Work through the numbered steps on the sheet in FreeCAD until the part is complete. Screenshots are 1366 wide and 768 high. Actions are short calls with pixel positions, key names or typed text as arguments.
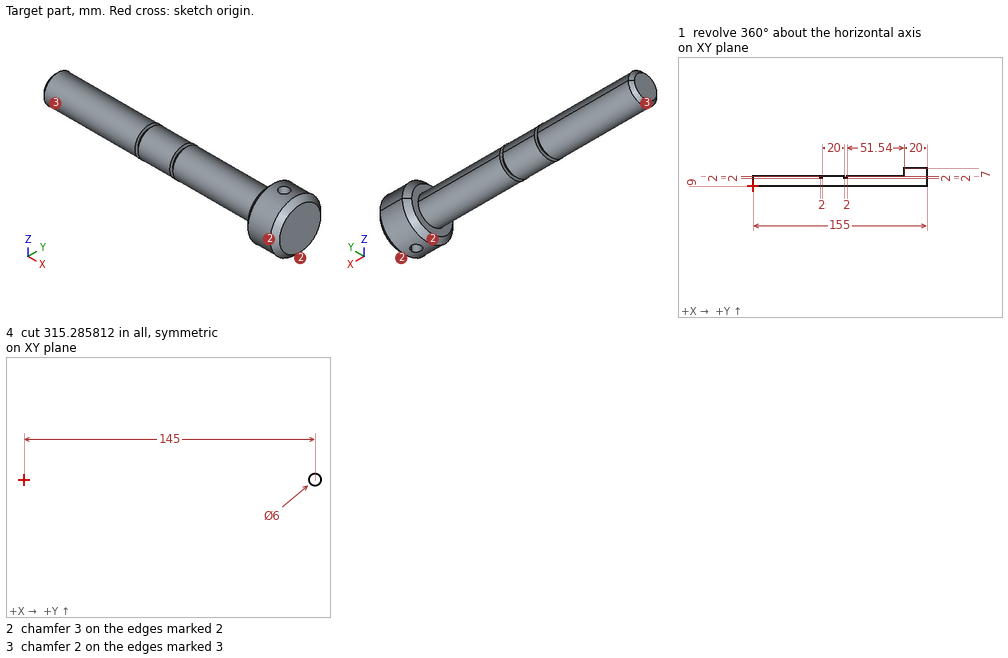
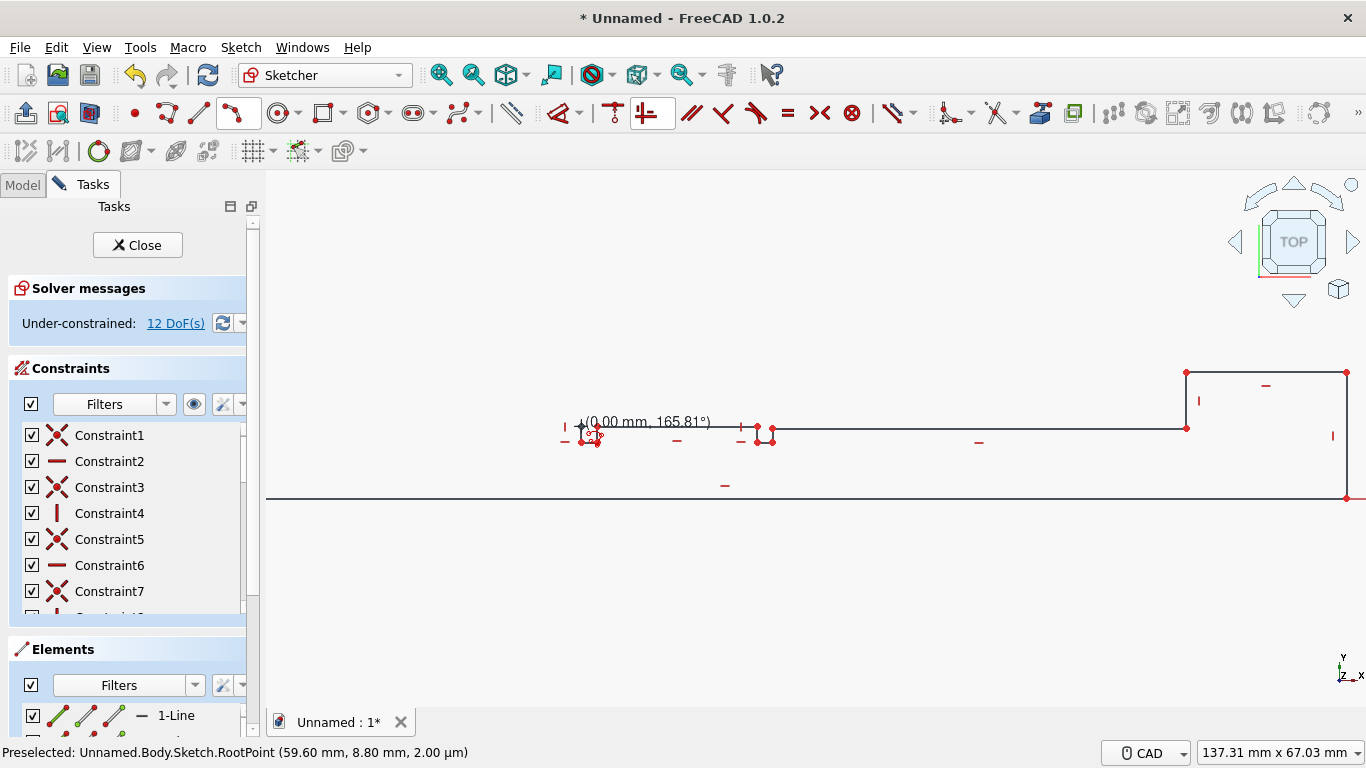
scroll(774, 443, down, 3)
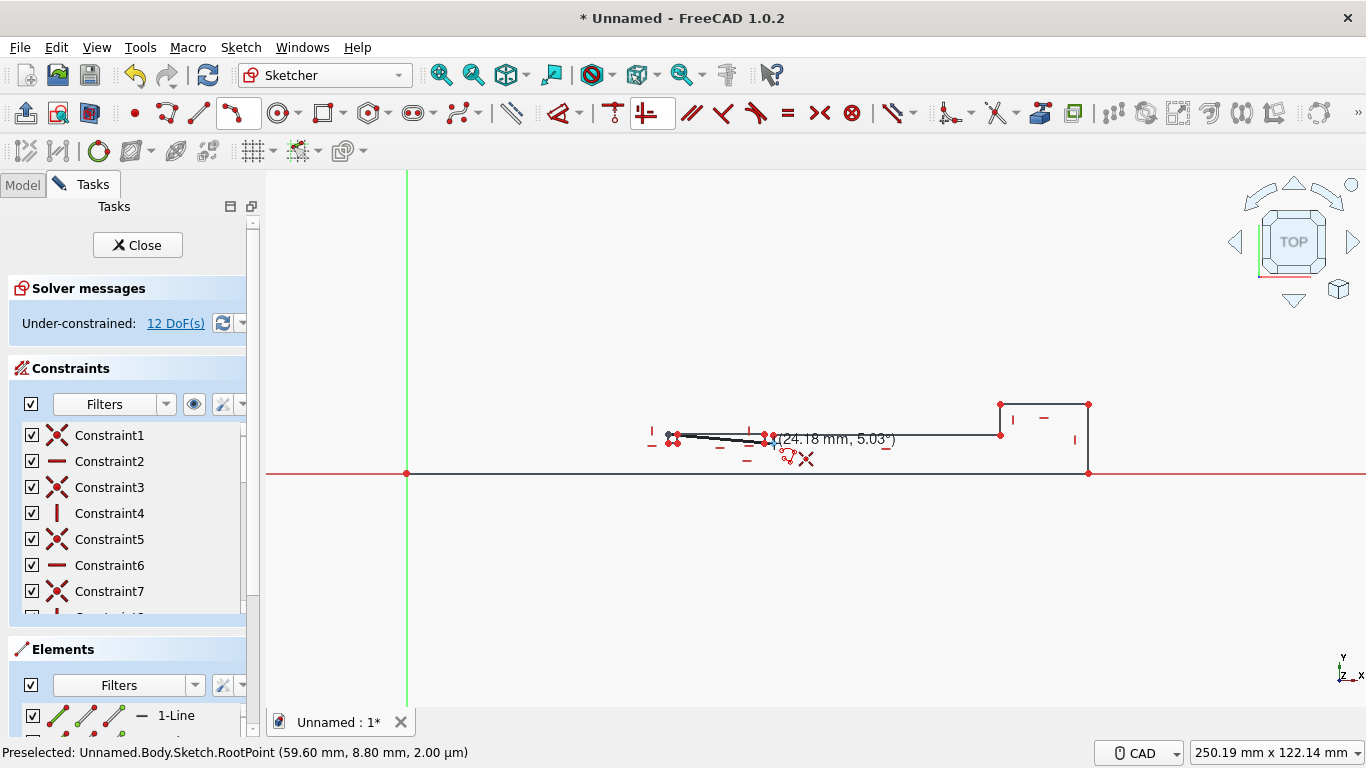
click(416, 434)
click(407, 474)
key(Escape)
key(Escape)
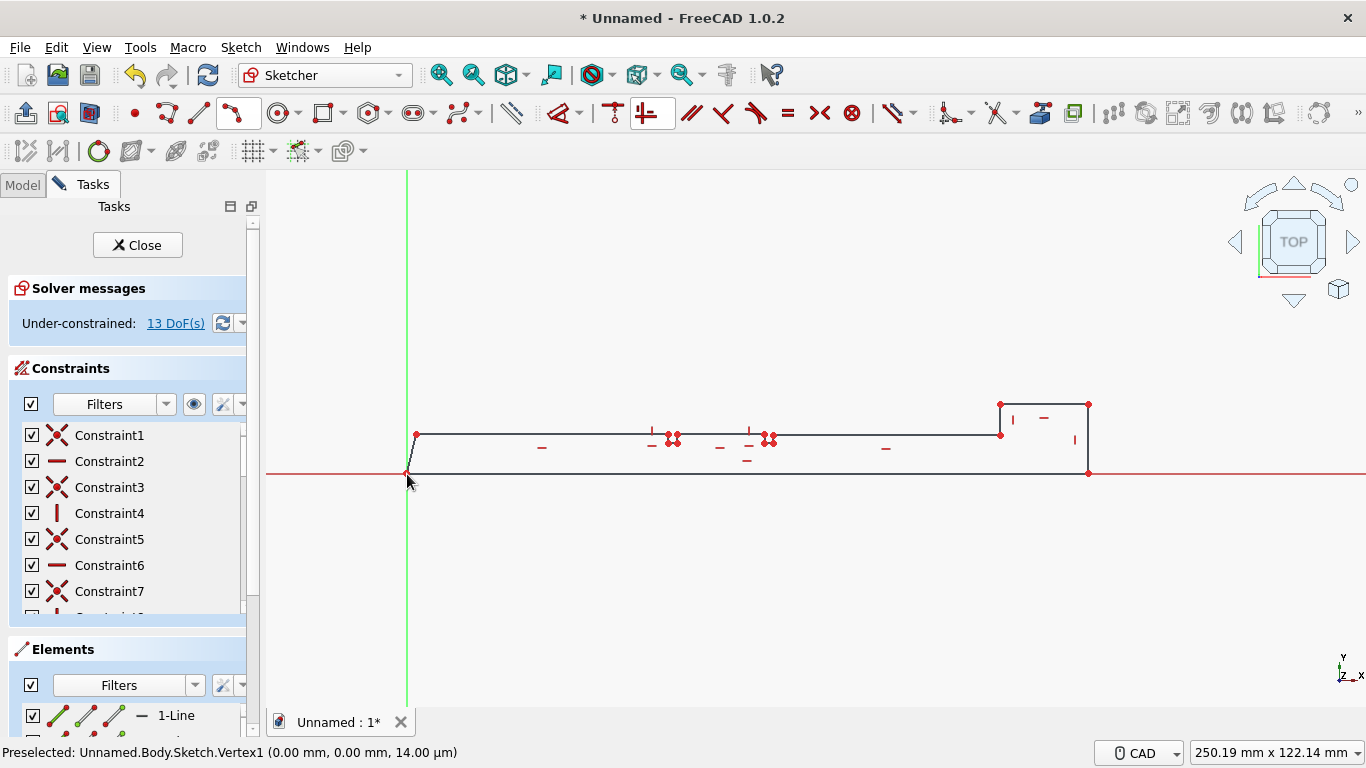
click(410, 462)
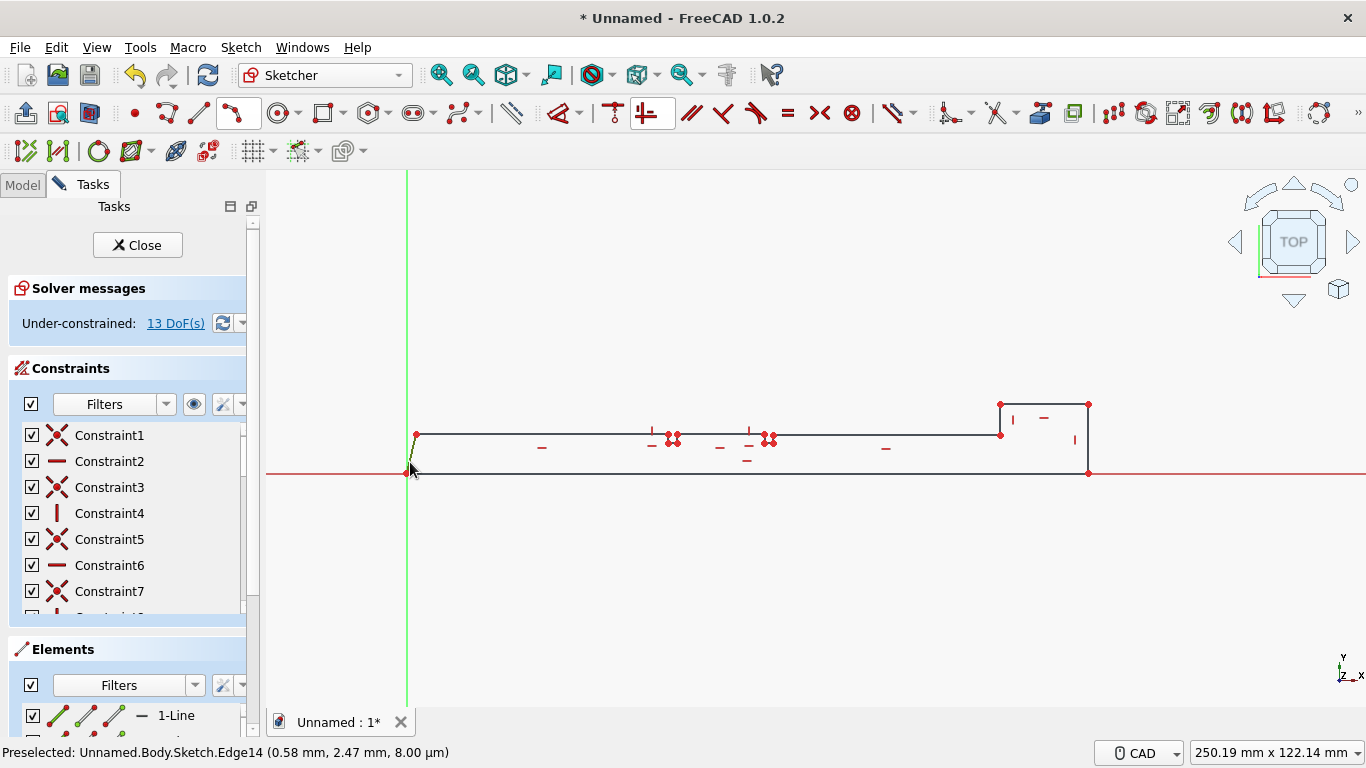
click(670, 114)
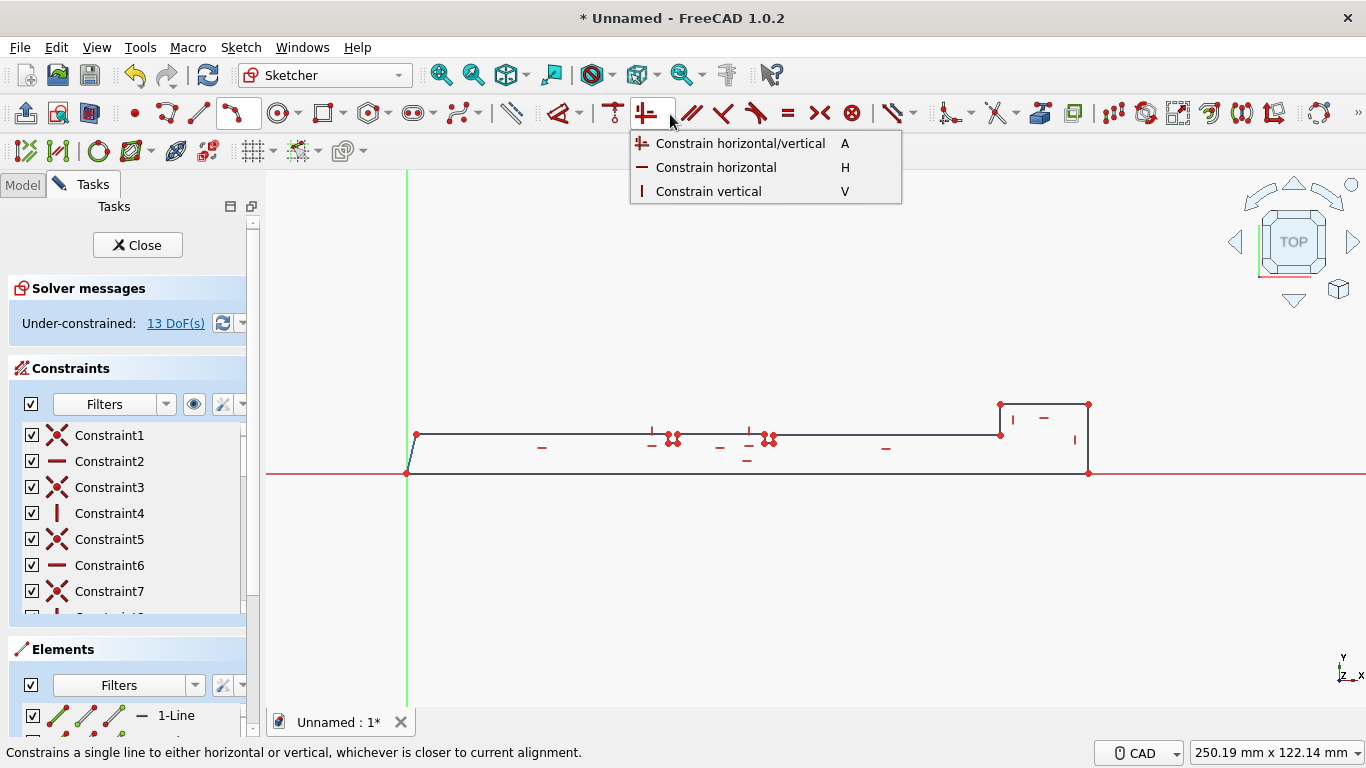
click(766, 191)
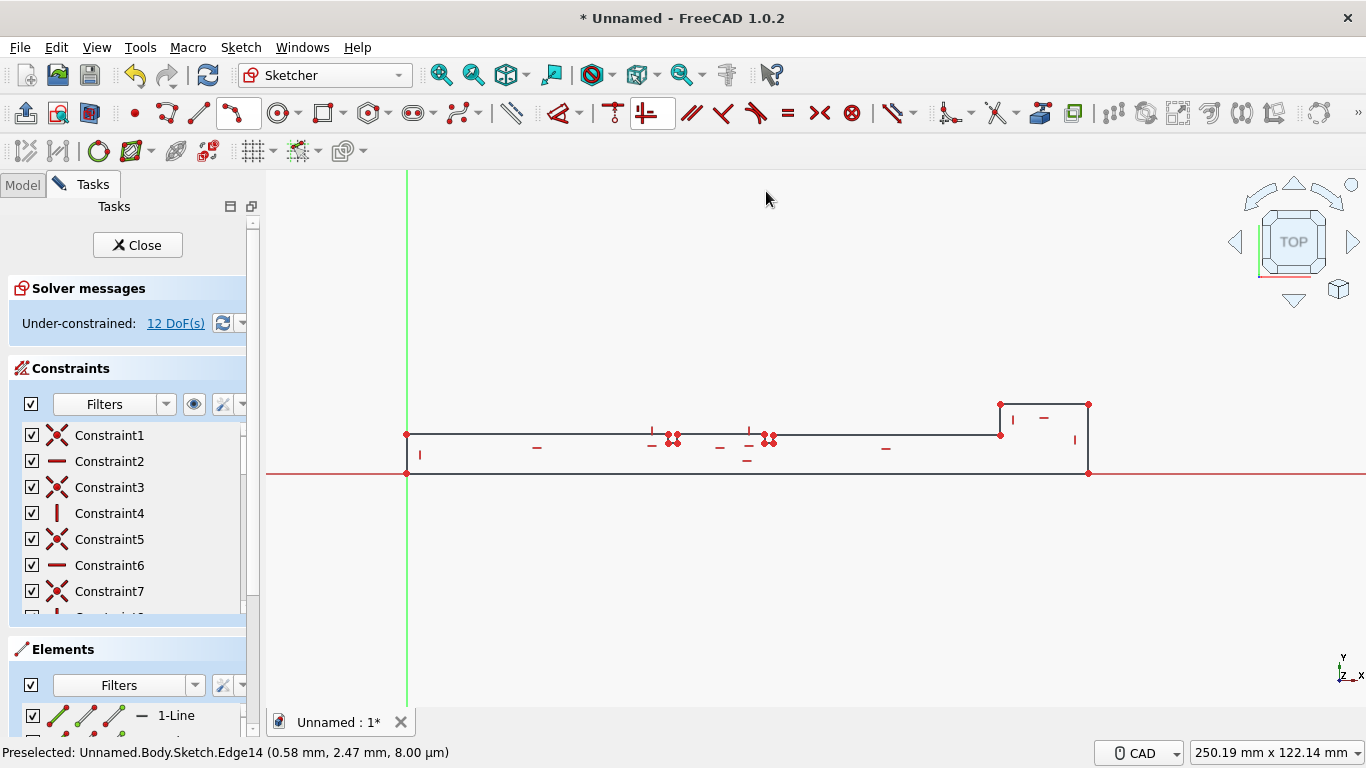
click(558, 114)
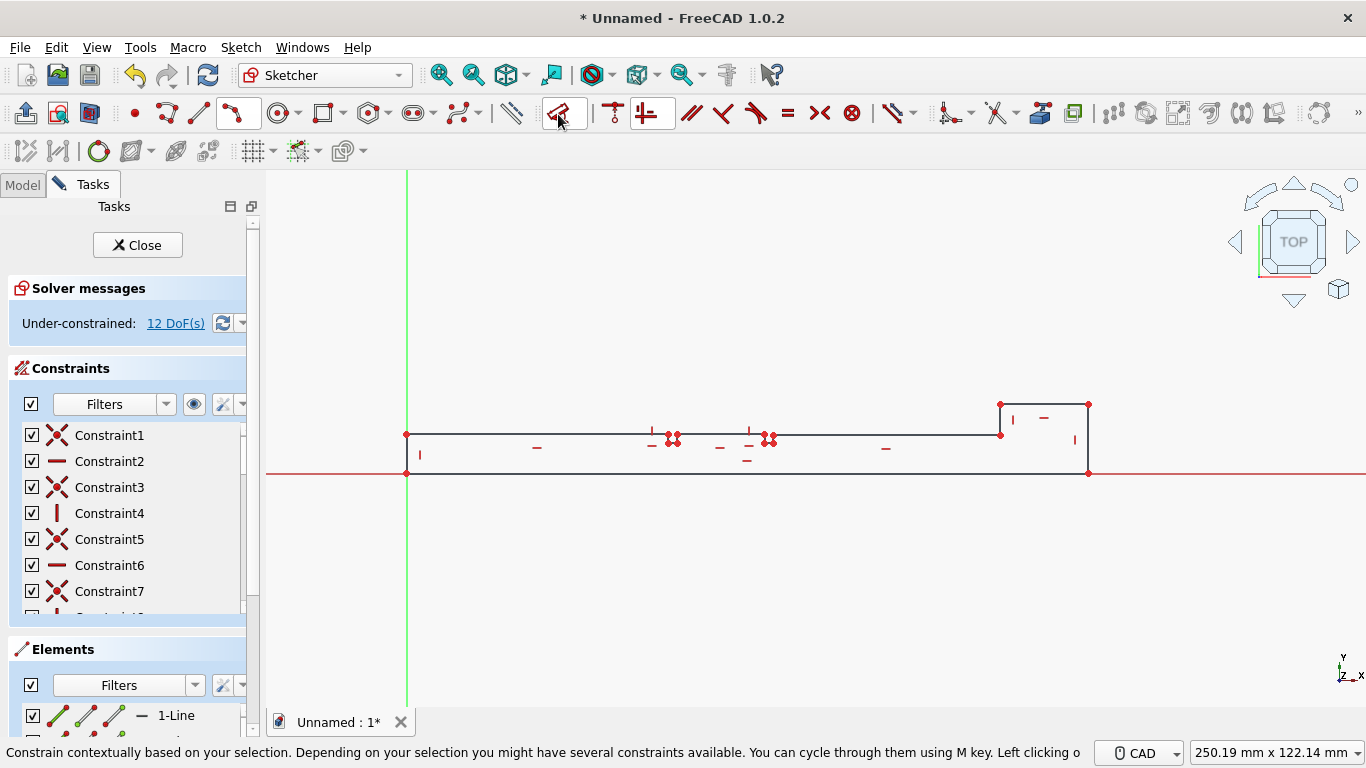
scroll(1000, 414, up, 2)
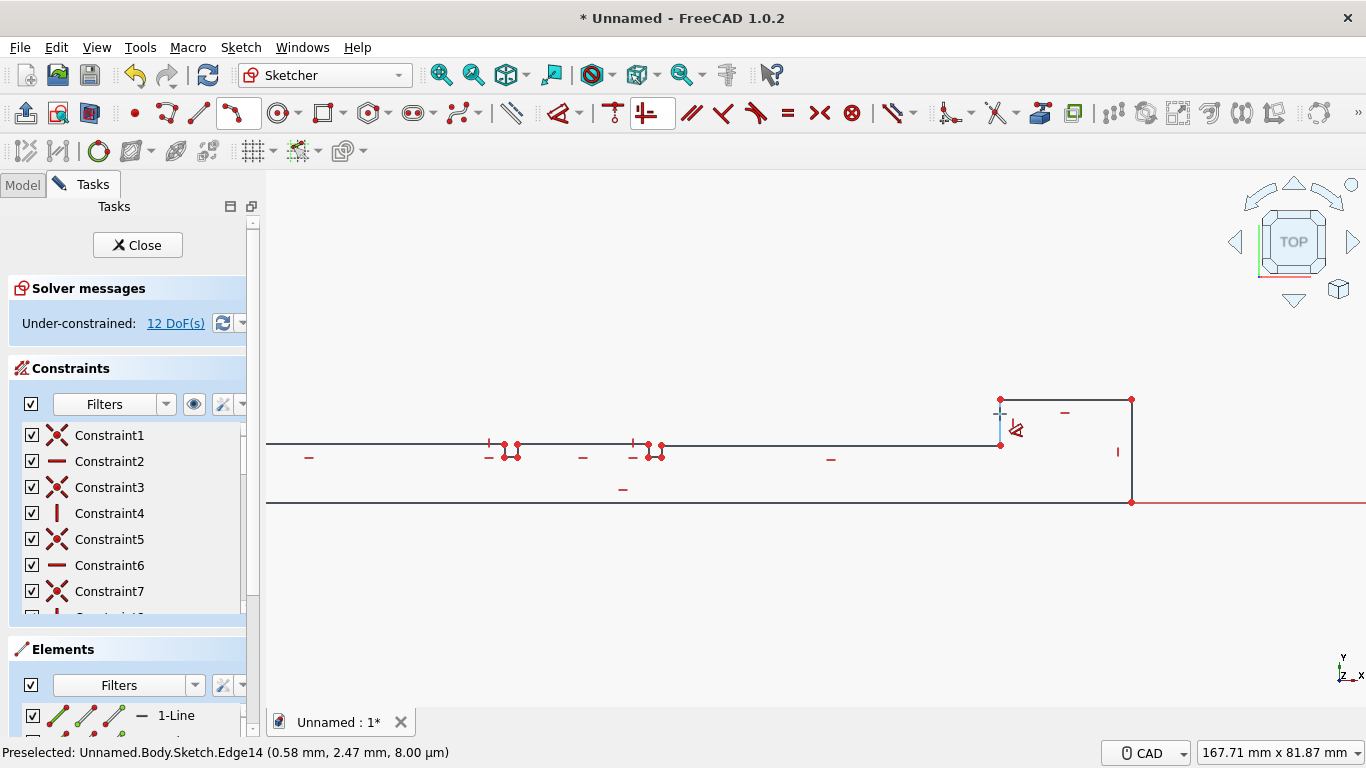
click(1000, 413)
click(1034, 423)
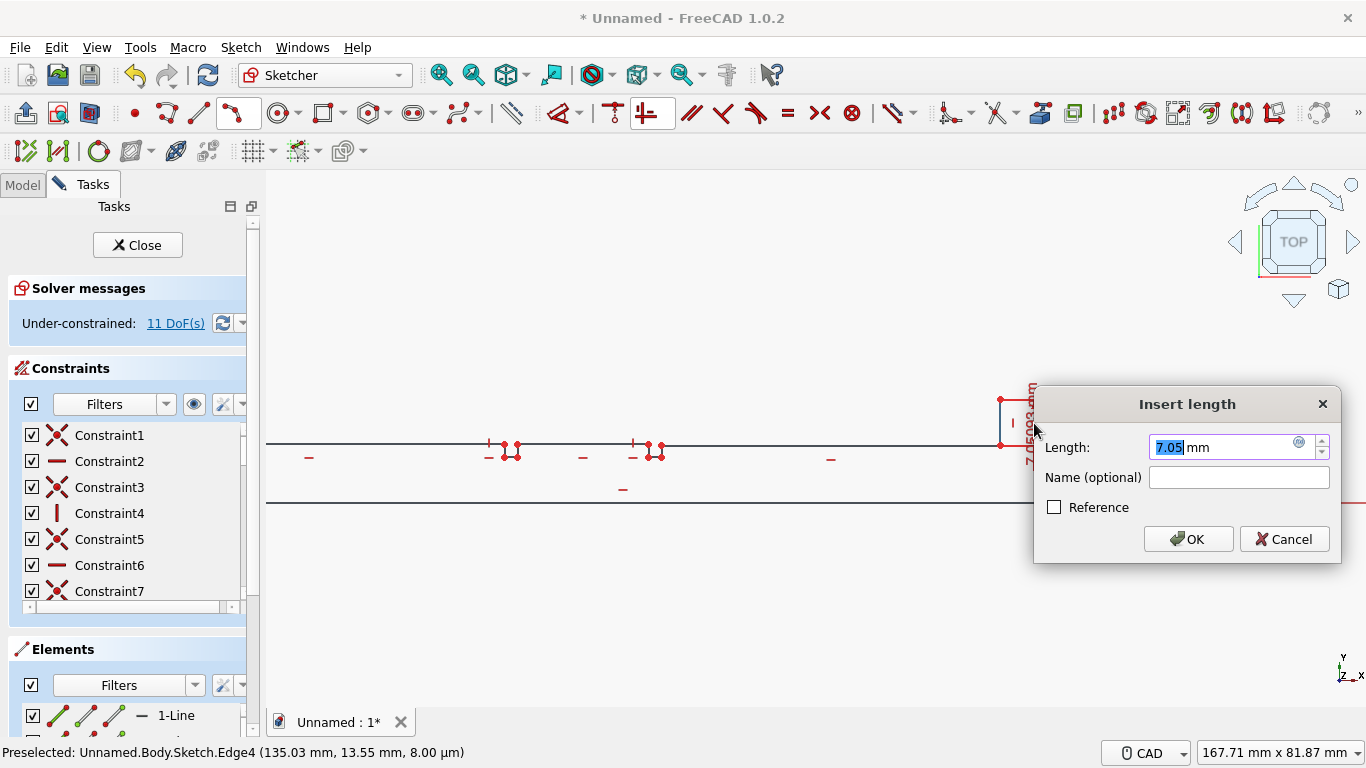
text(7)
key(Return)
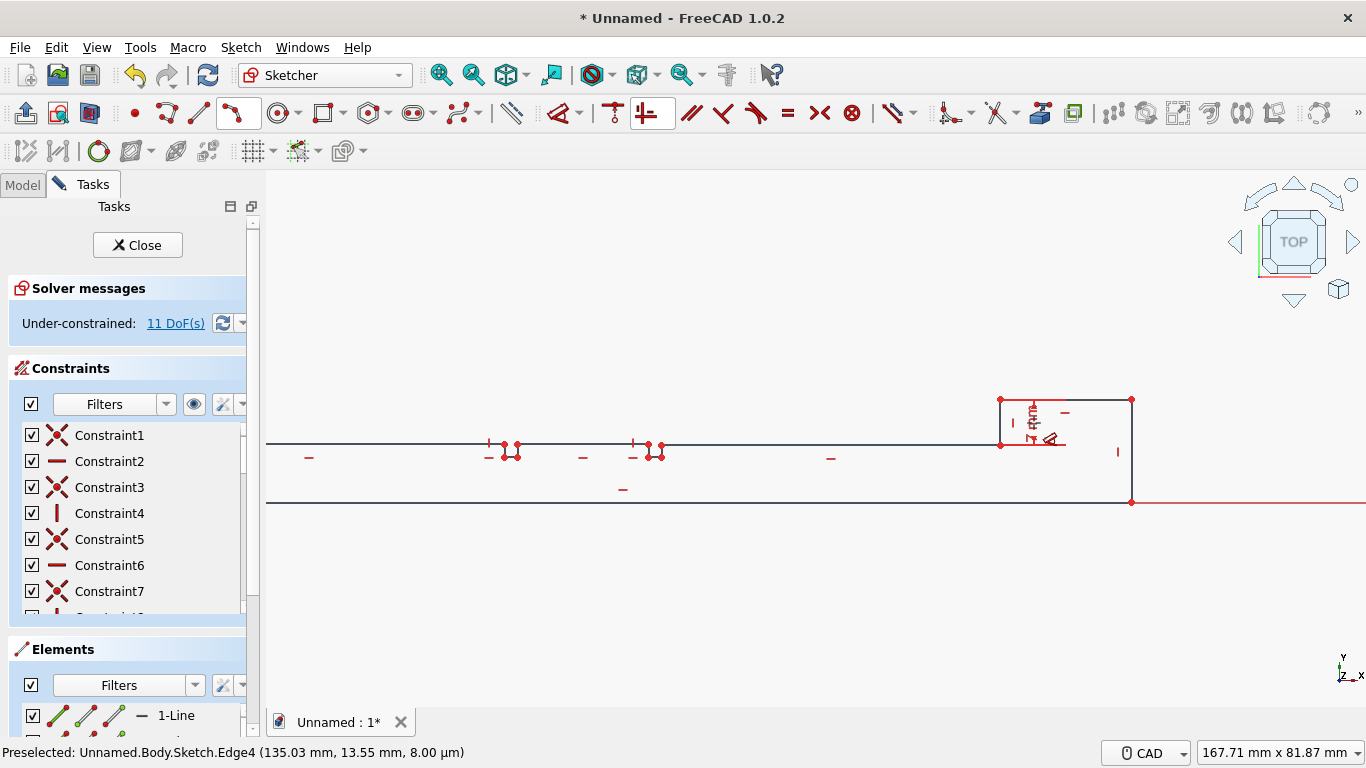
scroll(662, 451, up, 6)